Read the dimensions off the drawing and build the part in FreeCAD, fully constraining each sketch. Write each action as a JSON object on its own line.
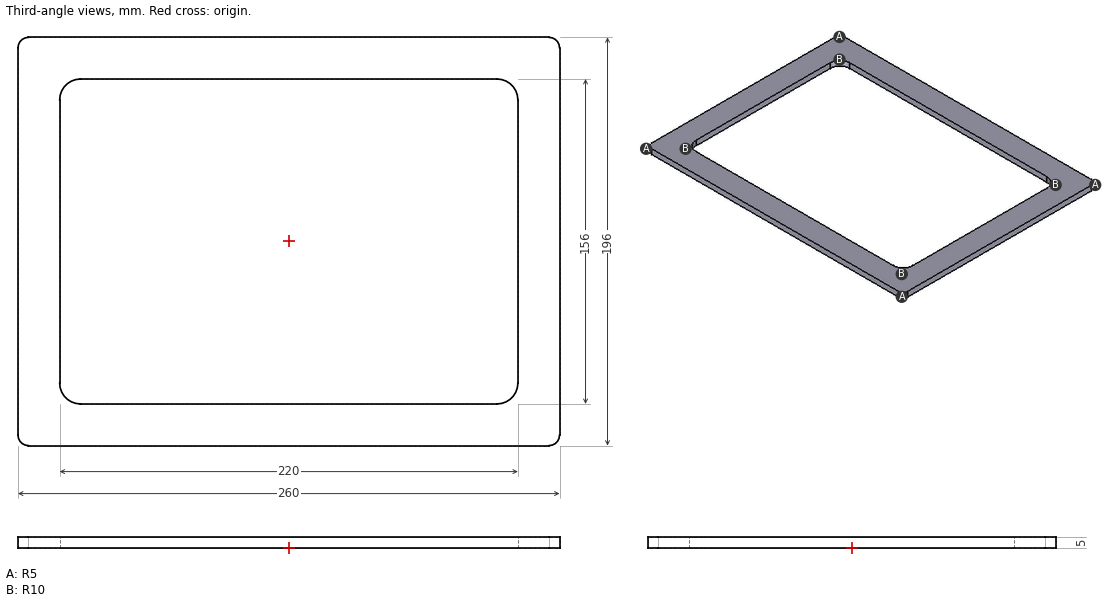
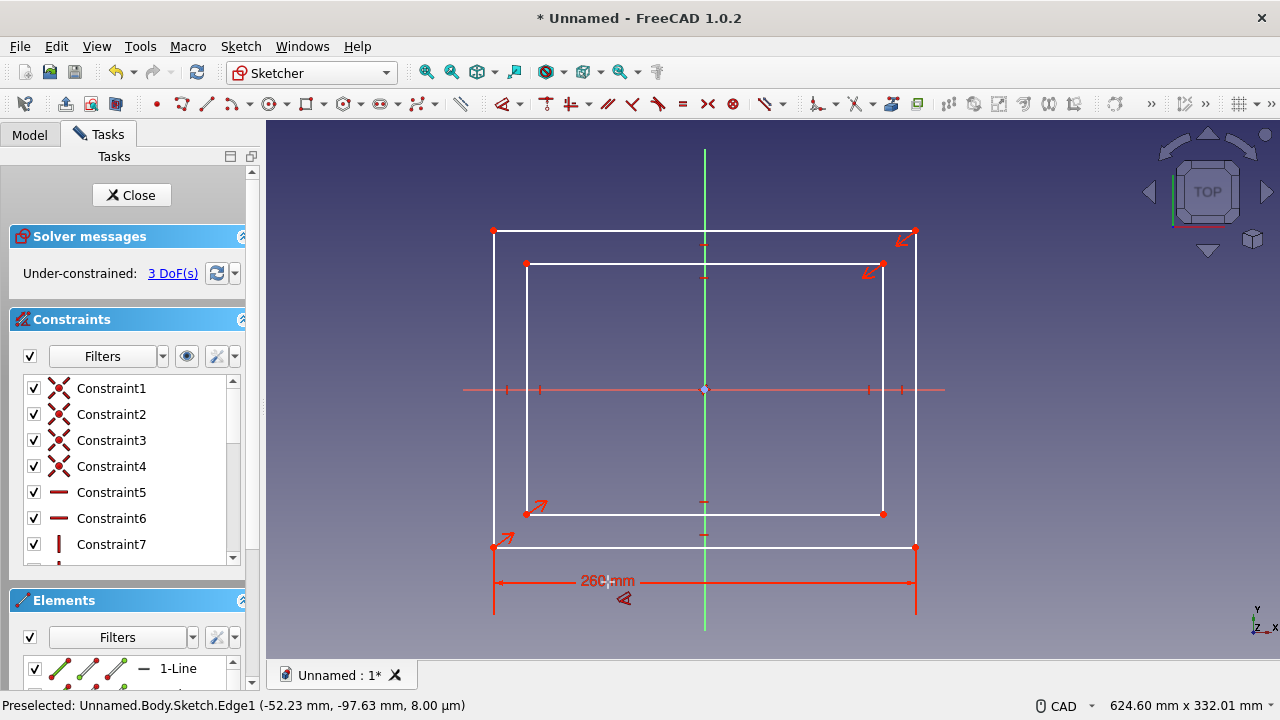
{"action": "left_click", "coordinate": [916, 453]}
{"action": "left_click", "coordinate": [950, 317]}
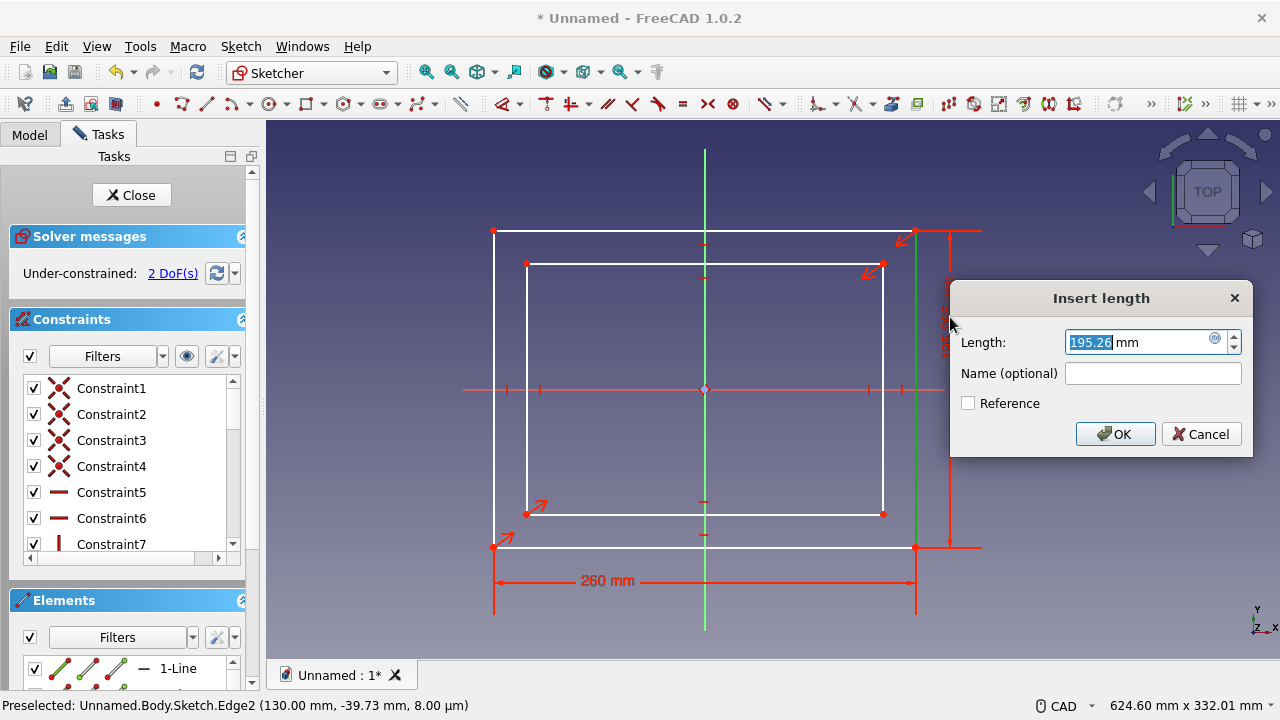
{"action": "type", "text": "196"}
{"action": "key", "text": "Return"}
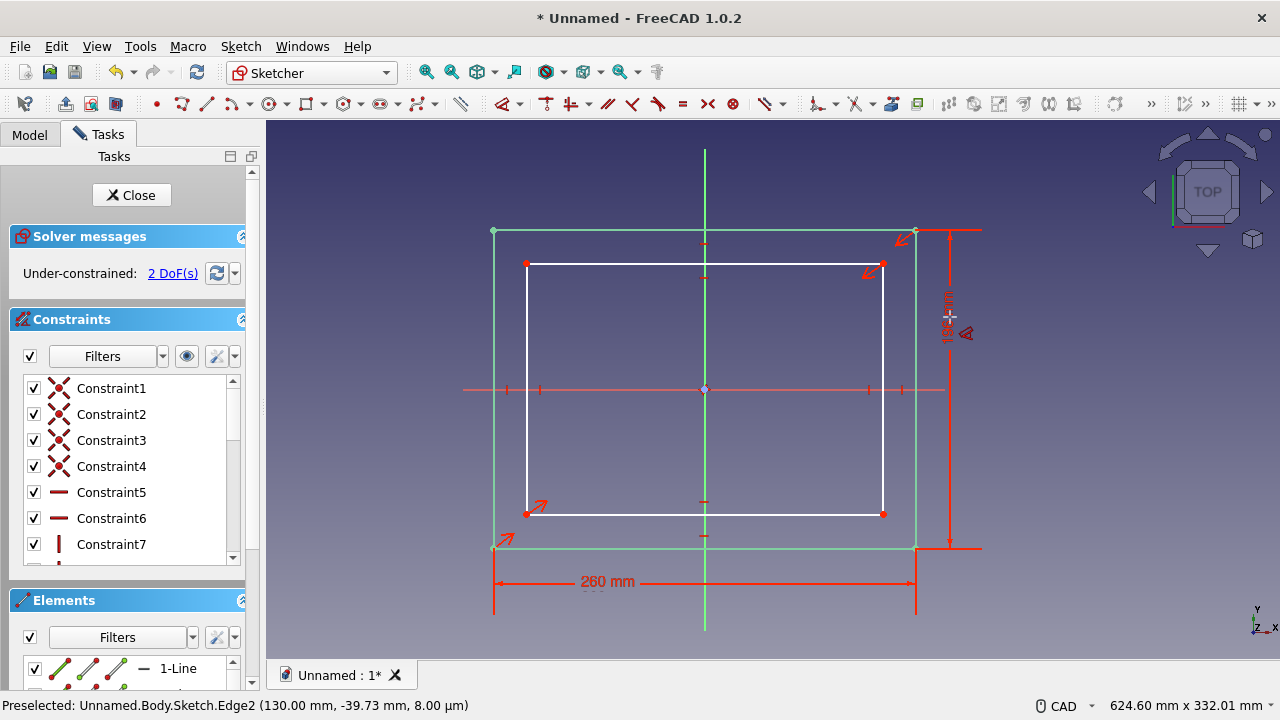
{"action": "left_click", "coordinate": [634, 515]}
{"action": "left_click", "coordinate": [623, 481]}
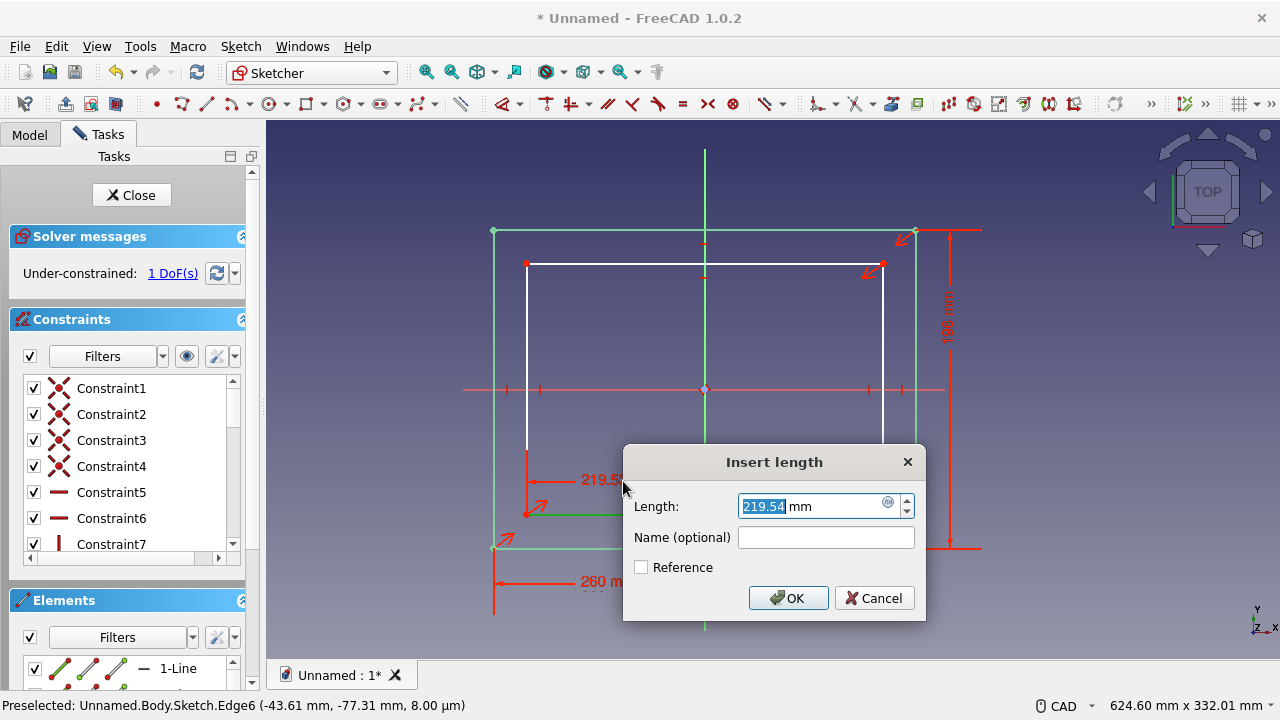
{"action": "type", "text": "220"}
{"action": "key", "text": "Return"}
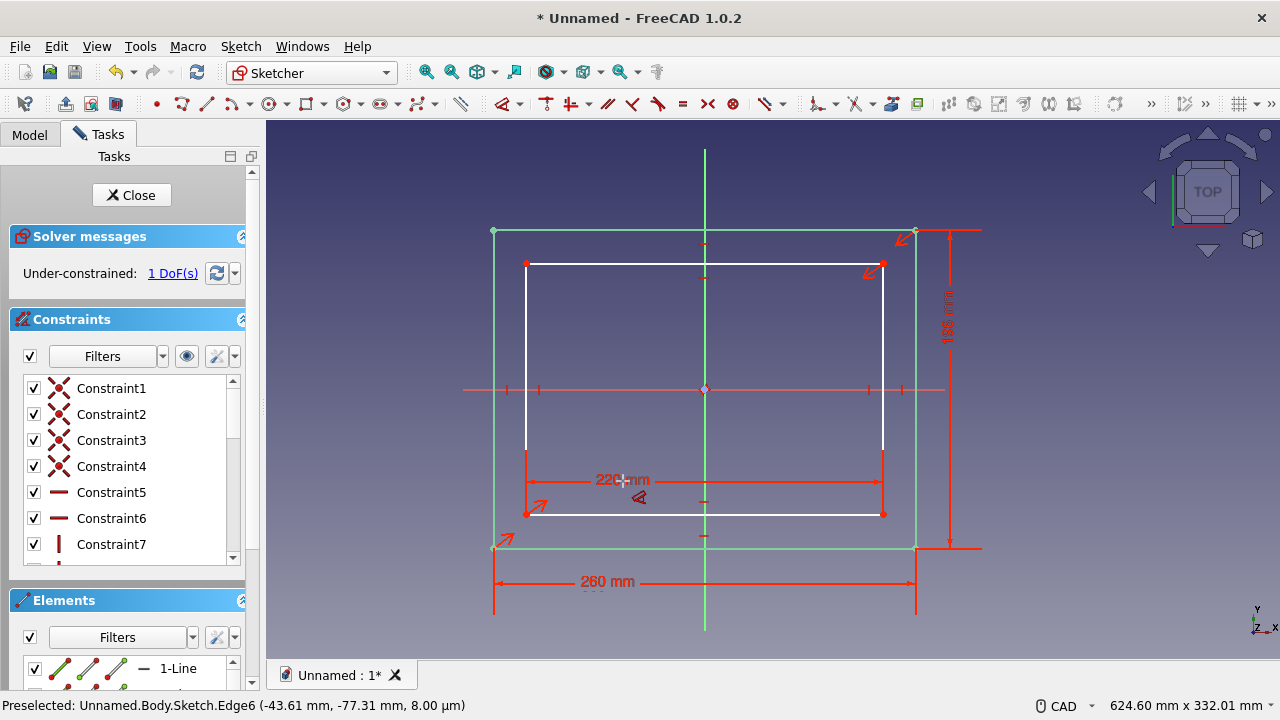
{"action": "left_click", "coordinate": [883, 440]}
{"action": "left_click", "coordinate": [849, 332]}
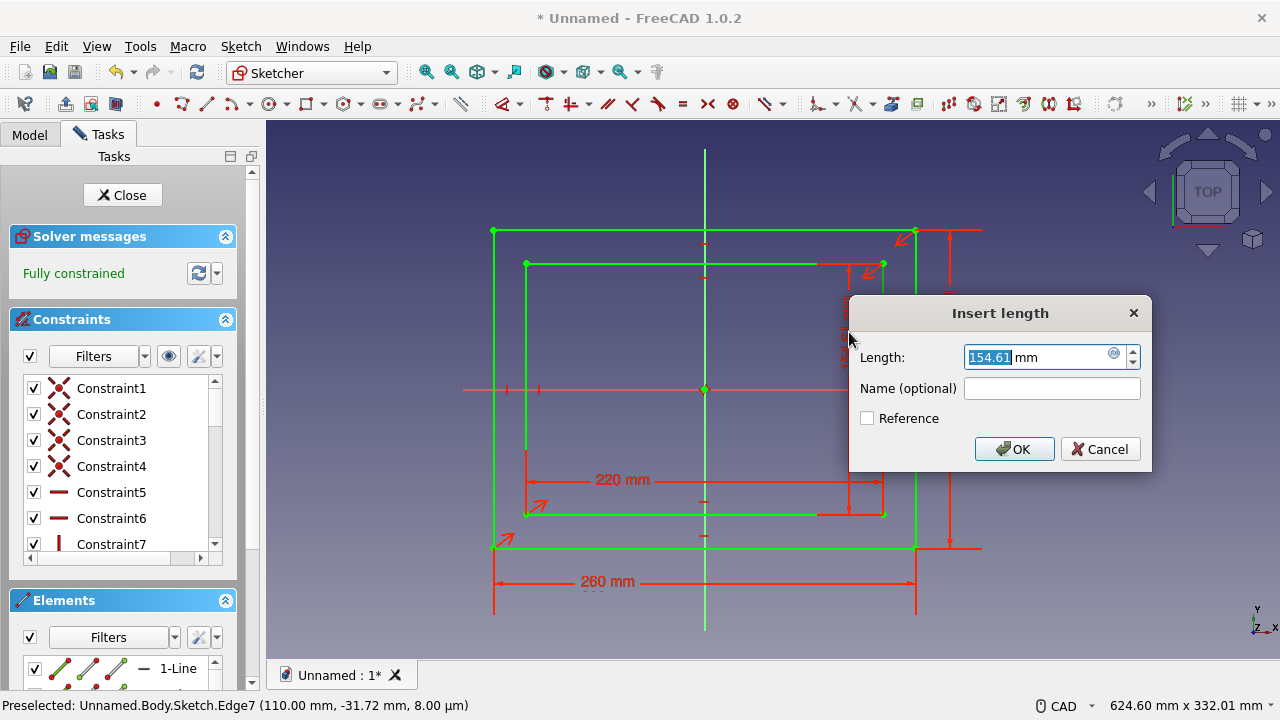
{"action": "type", "text": "156"}
{"action": "key", "text": "Return"}
{"action": "key", "text": "Escape"}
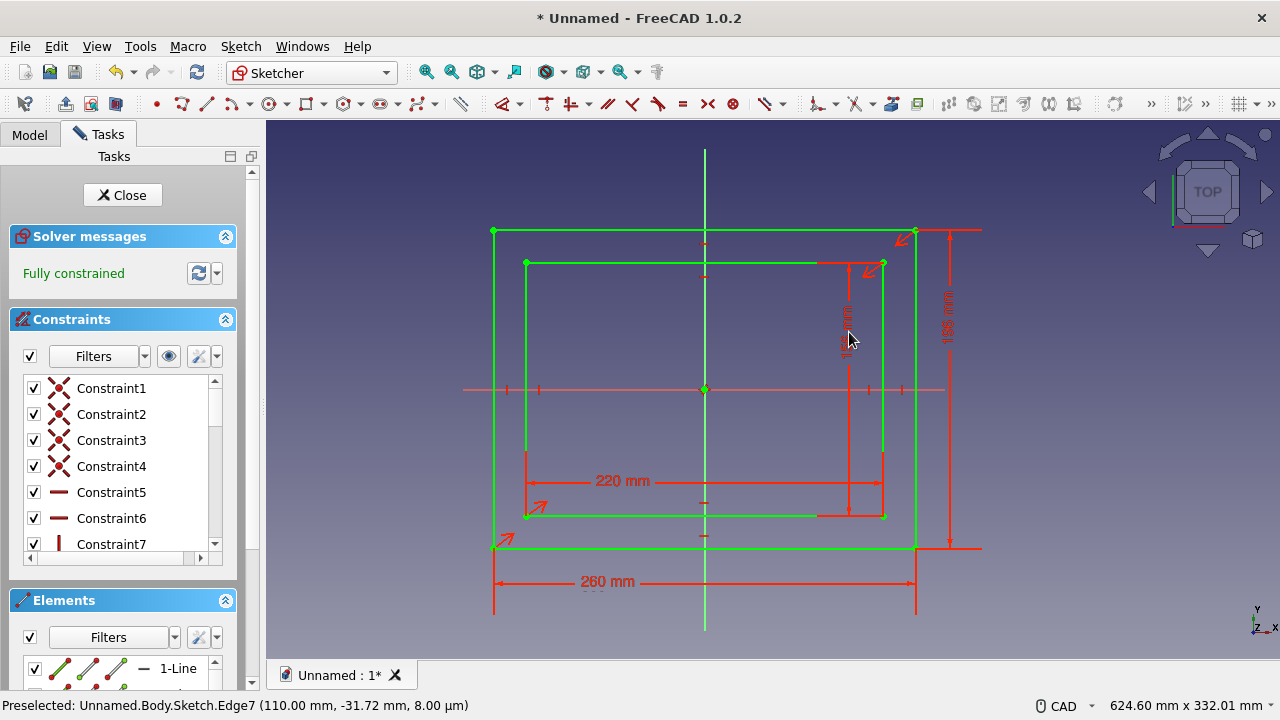
{"action": "left_click", "coordinate": [123, 195]}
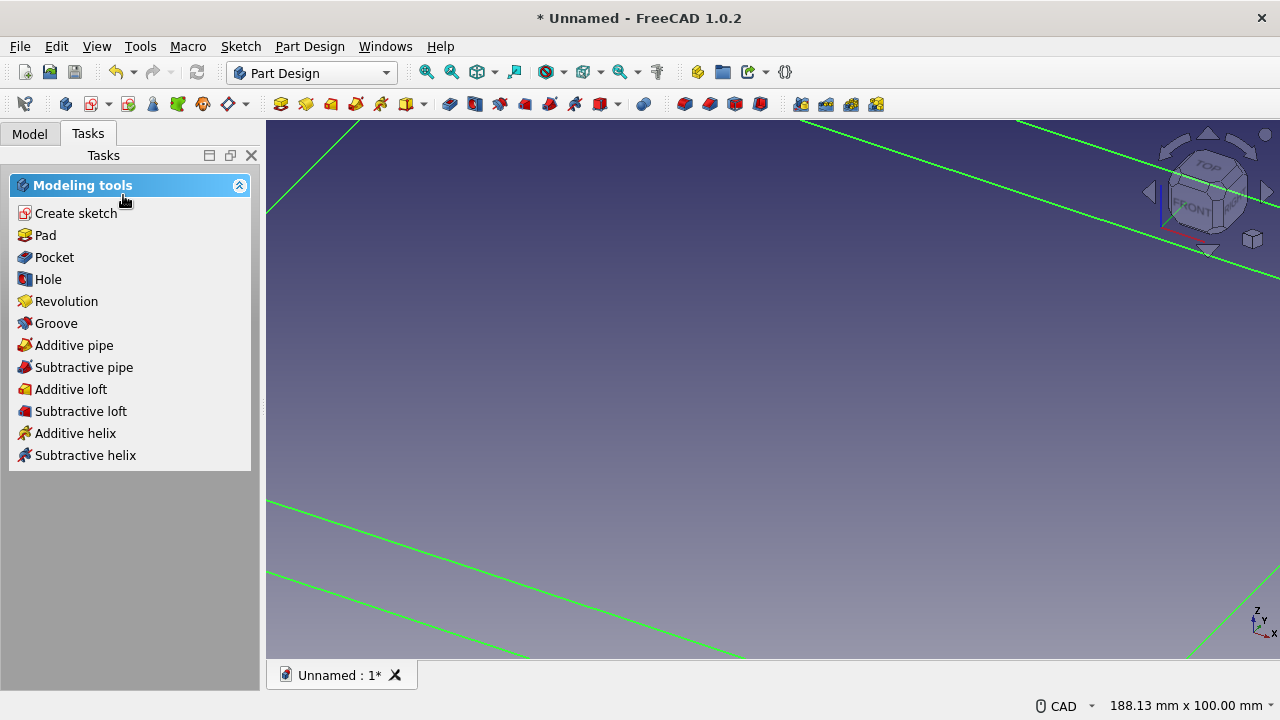
{"action": "left_click", "coordinate": [281, 104]}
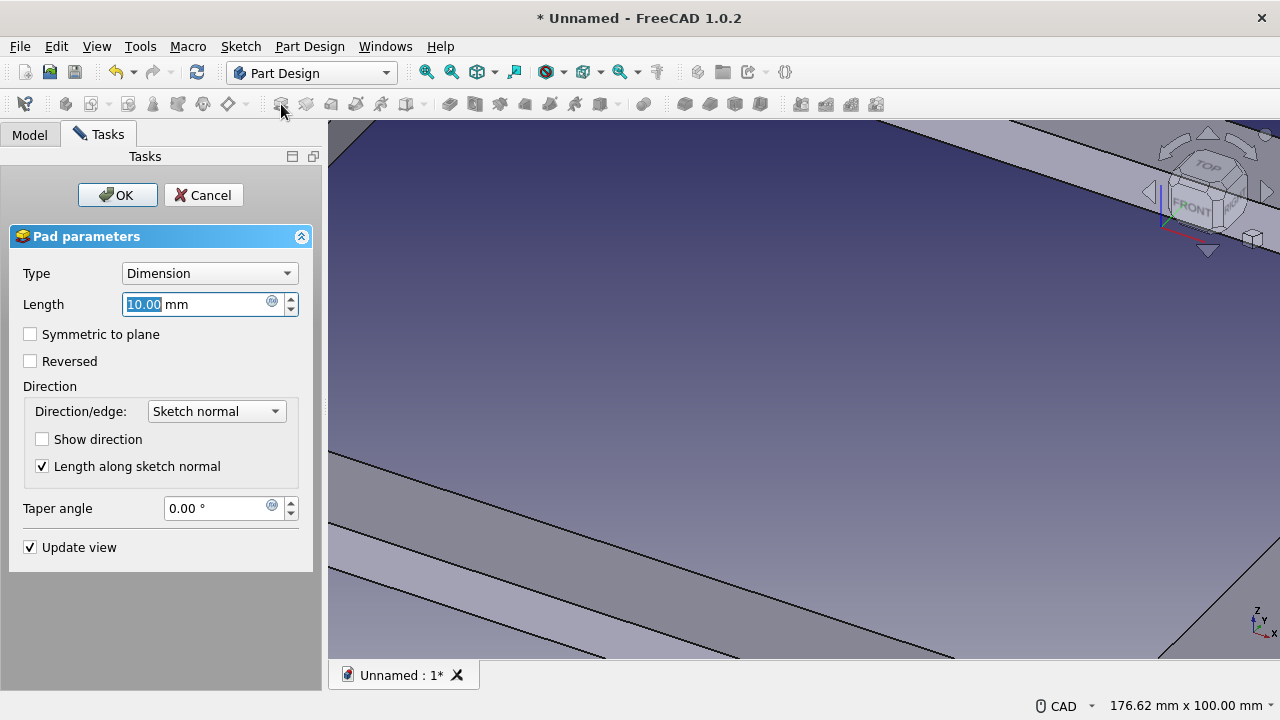
{"action": "type", "text": "5"}
{"action": "key", "text": "Tab"}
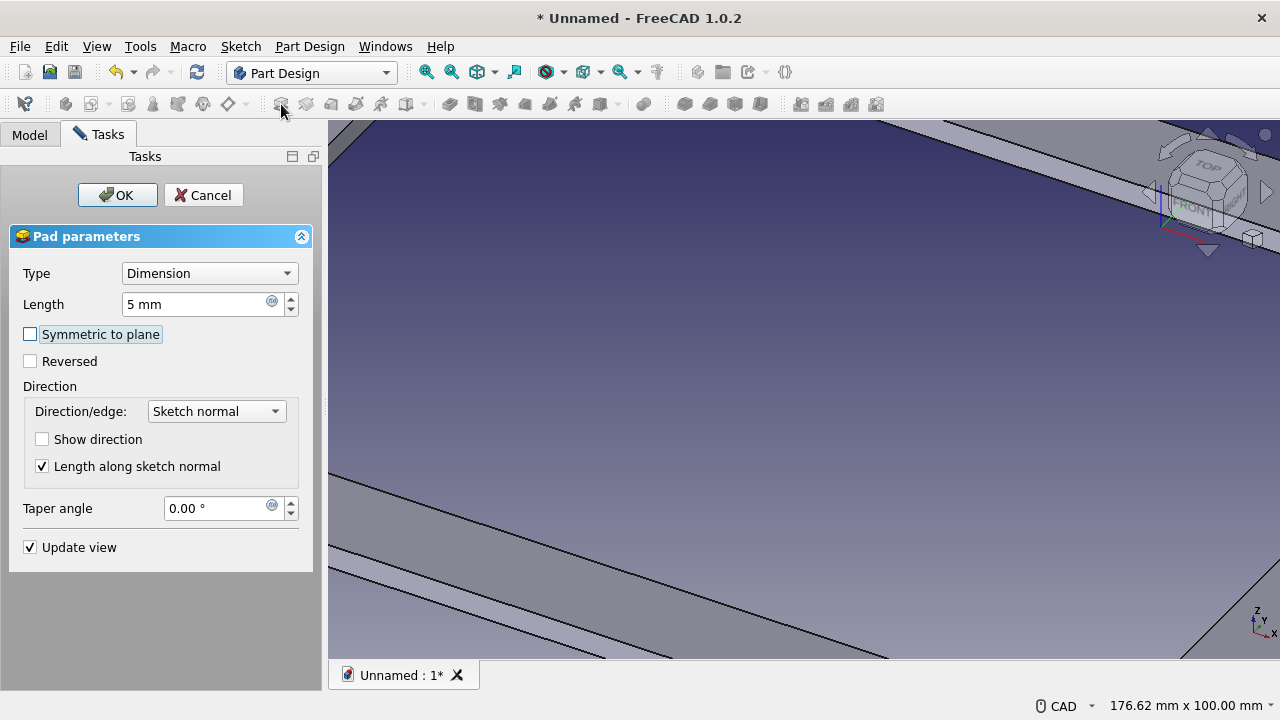
{"action": "left_click", "coordinate": [118, 195]}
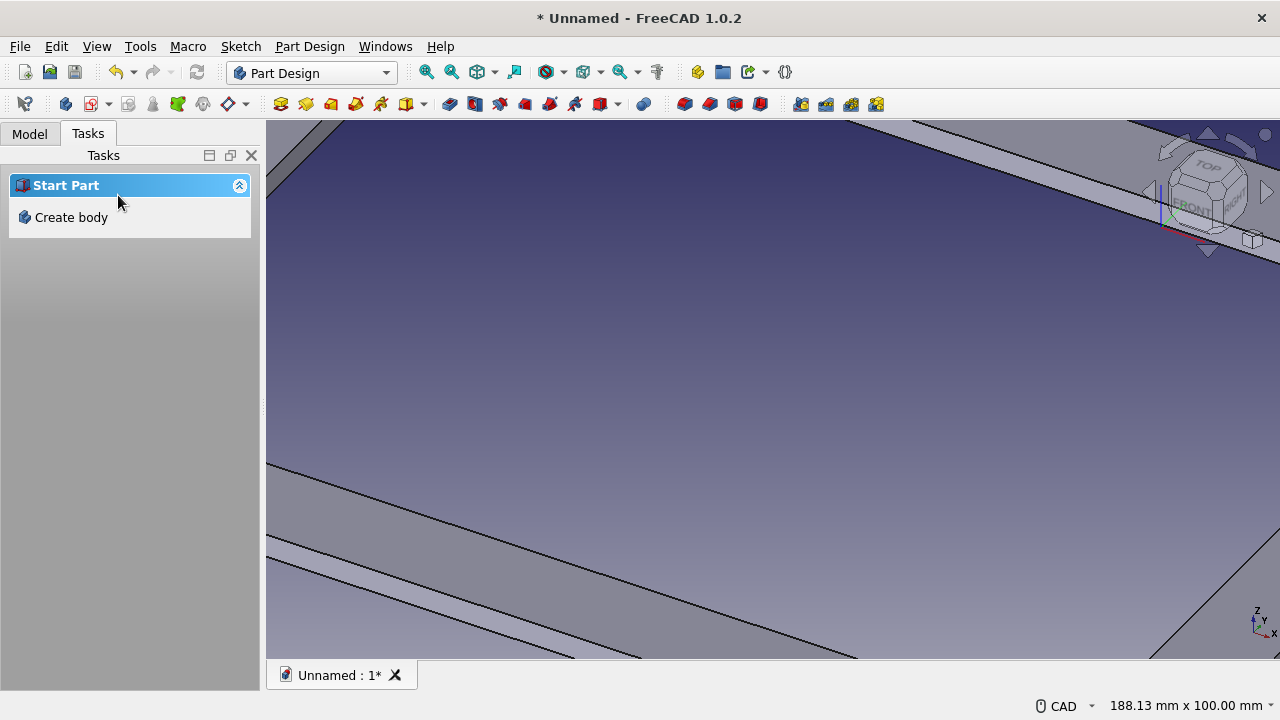
{"action": "left_click", "coordinate": [427, 72]}